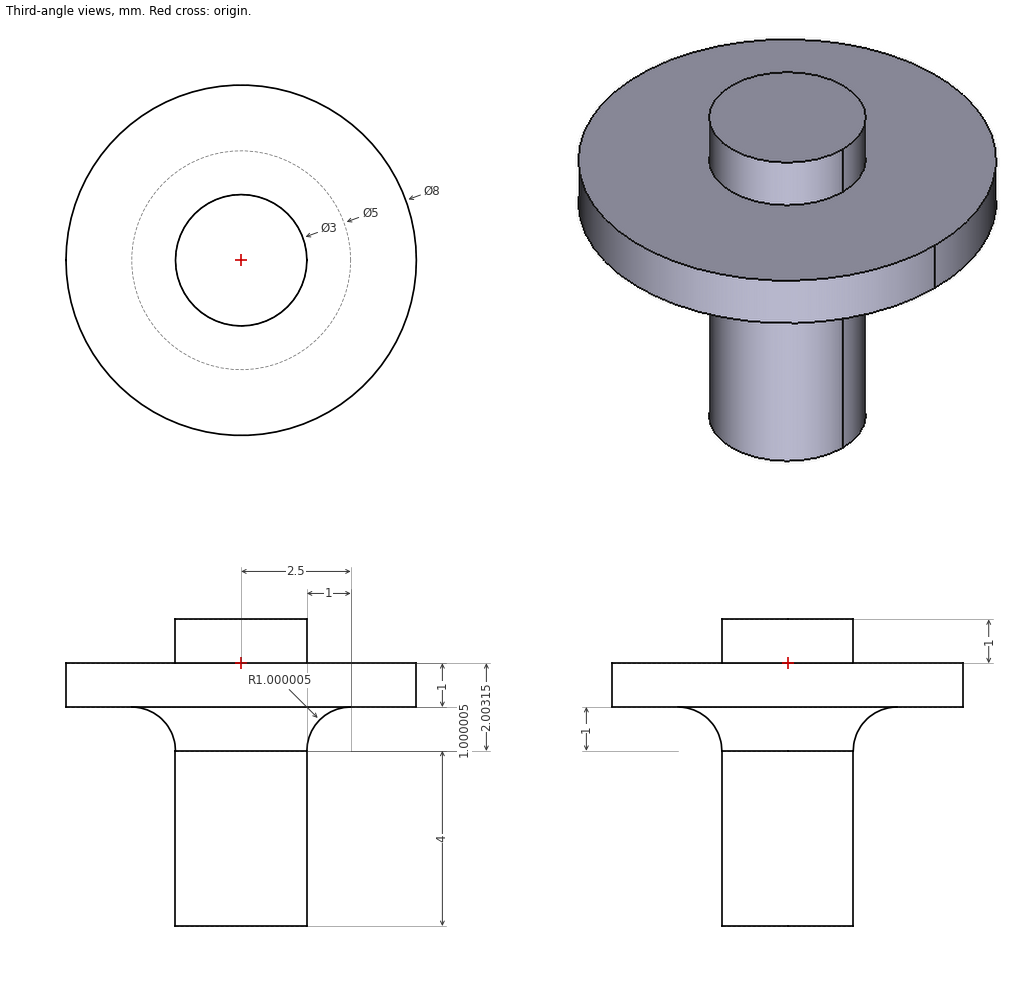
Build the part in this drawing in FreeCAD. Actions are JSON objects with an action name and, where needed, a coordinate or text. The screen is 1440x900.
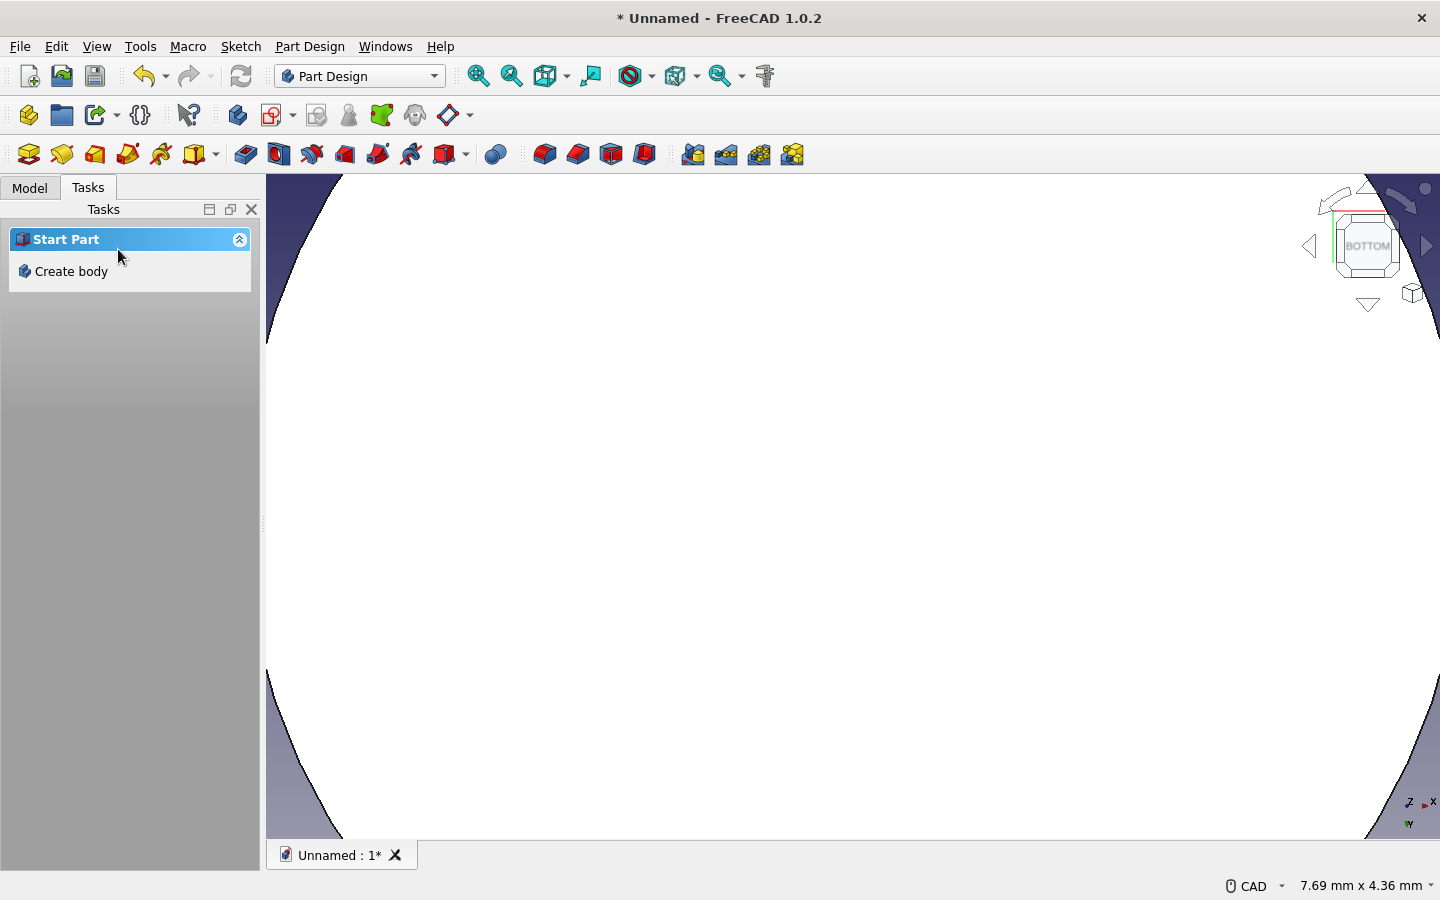
{"action": "left_click", "coordinate": [479, 76]}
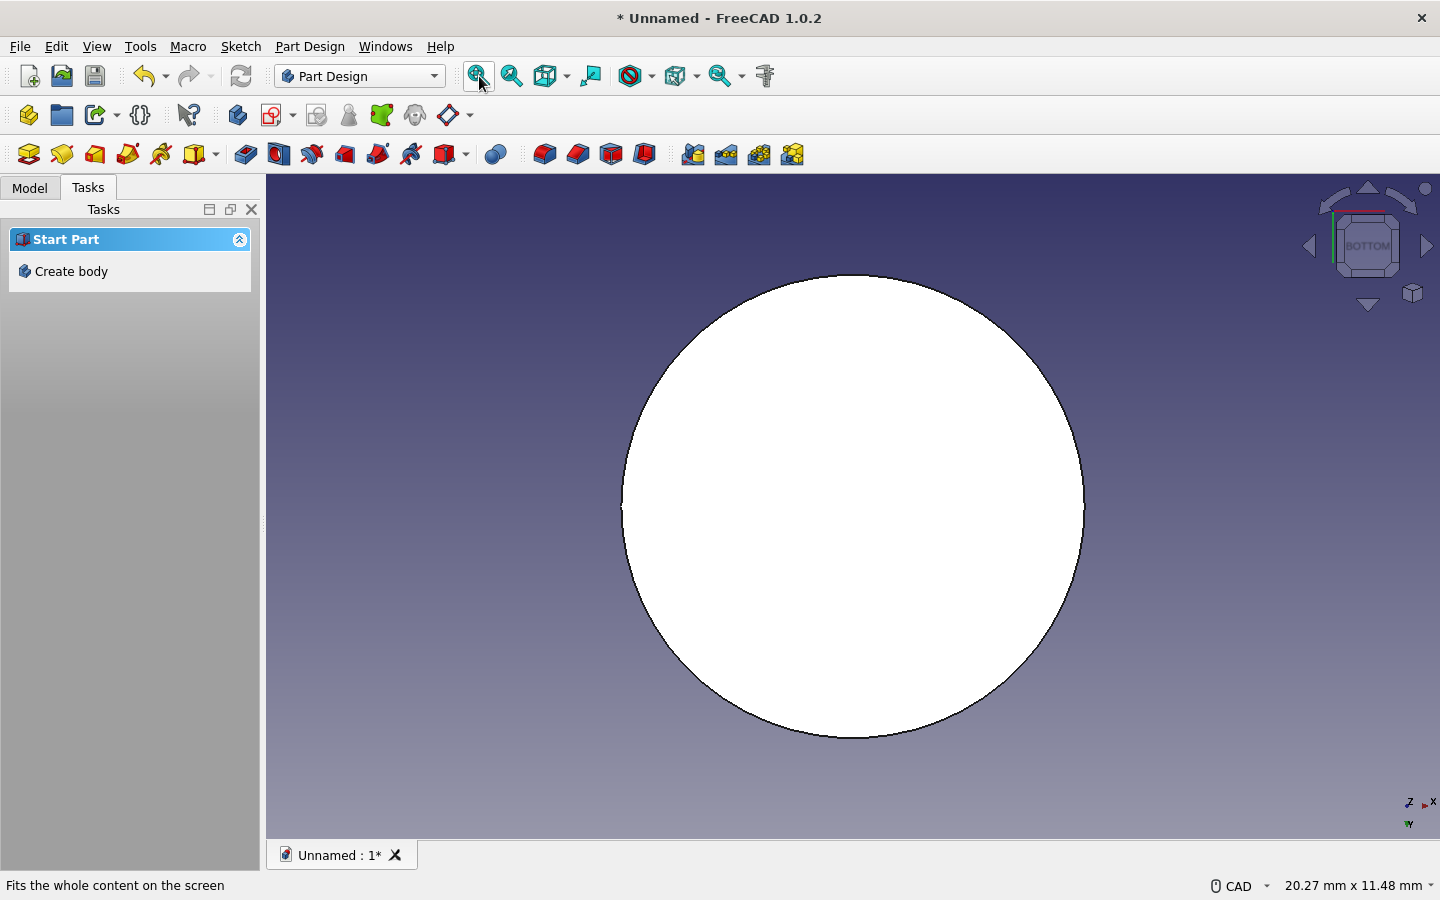
{"action": "left_click", "coordinate": [853, 505]}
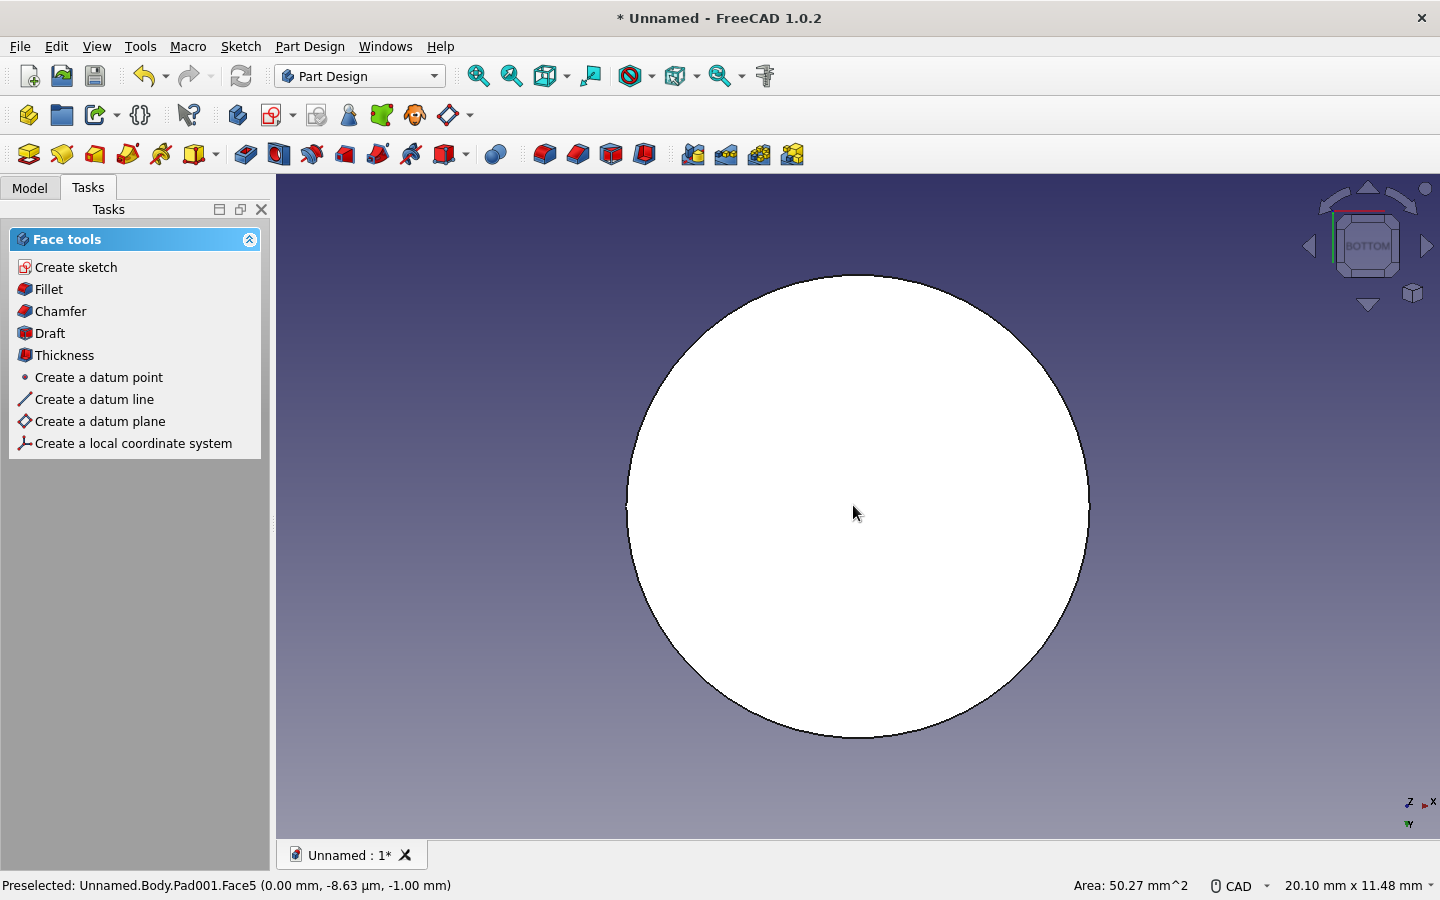
{"action": "left_click", "coordinate": [270, 116]}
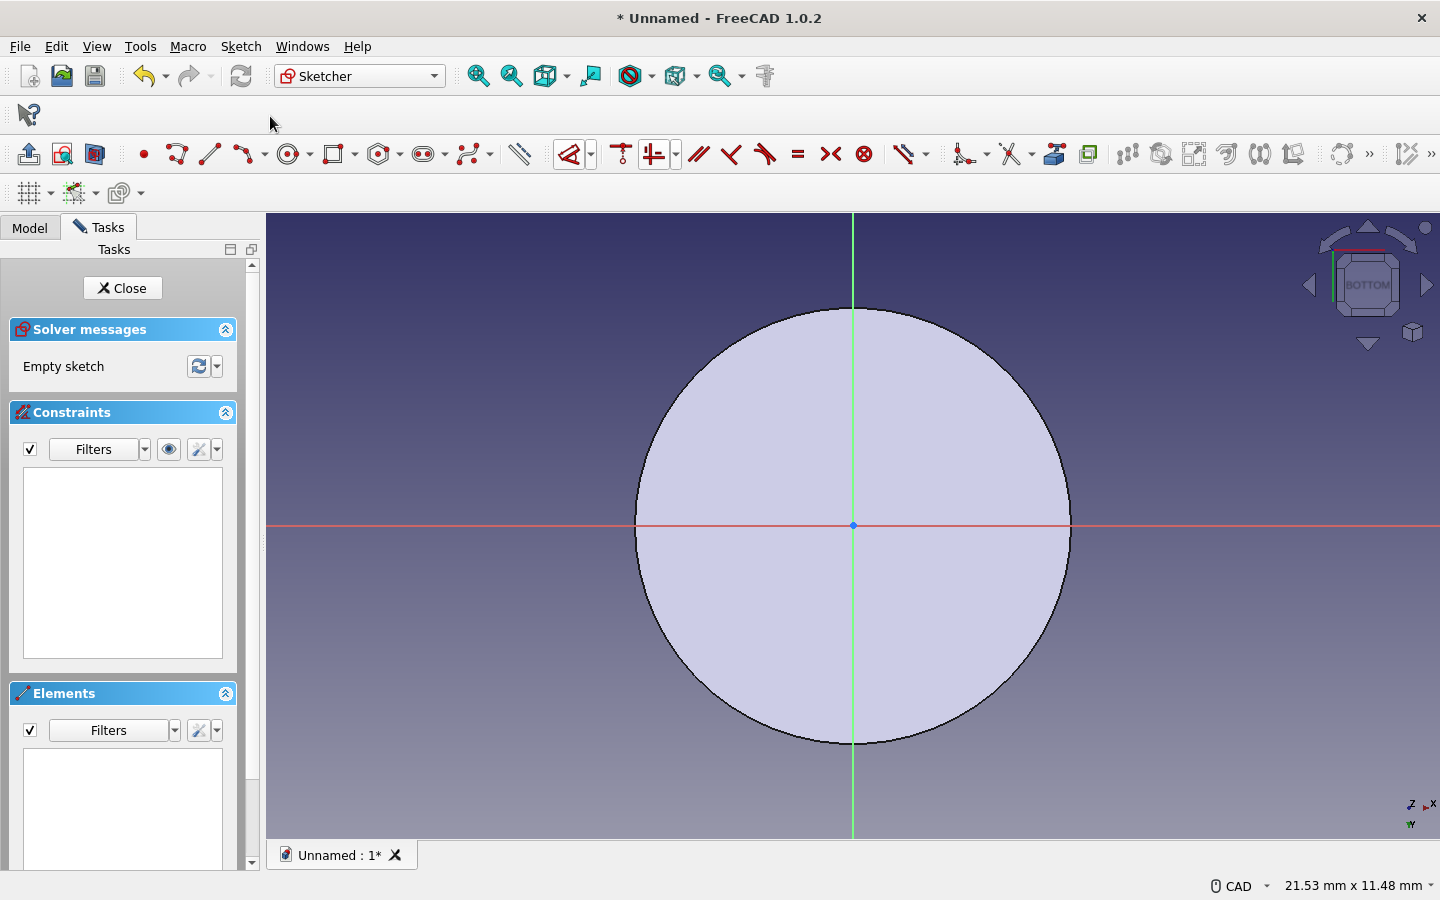
{"action": "scroll", "coordinate": [992, 526], "scroll_direction": "up", "scroll_amount": 2}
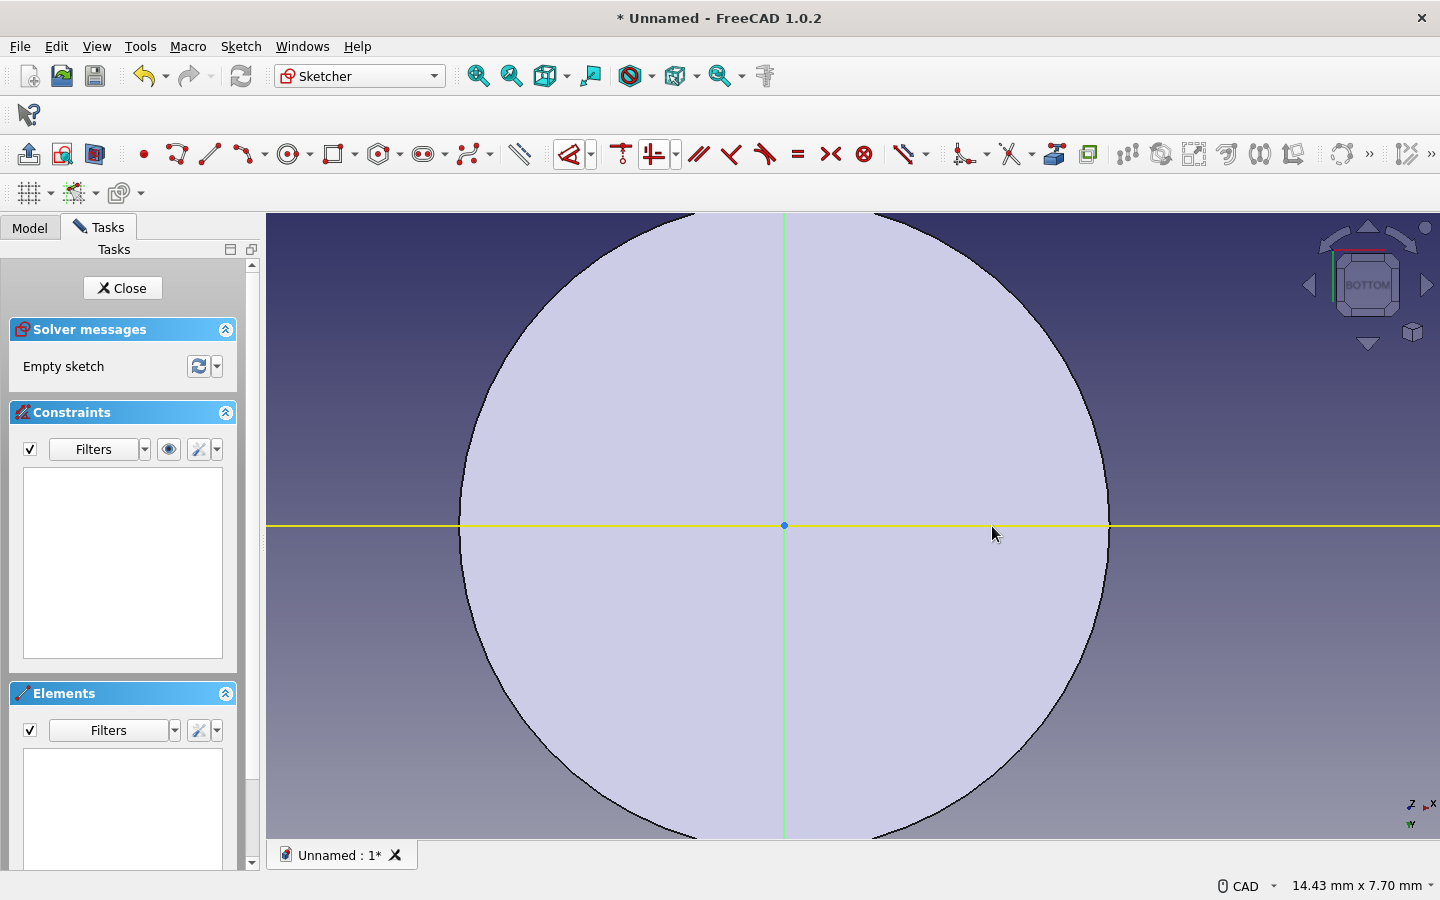
{"action": "left_click", "coordinate": [288, 154]}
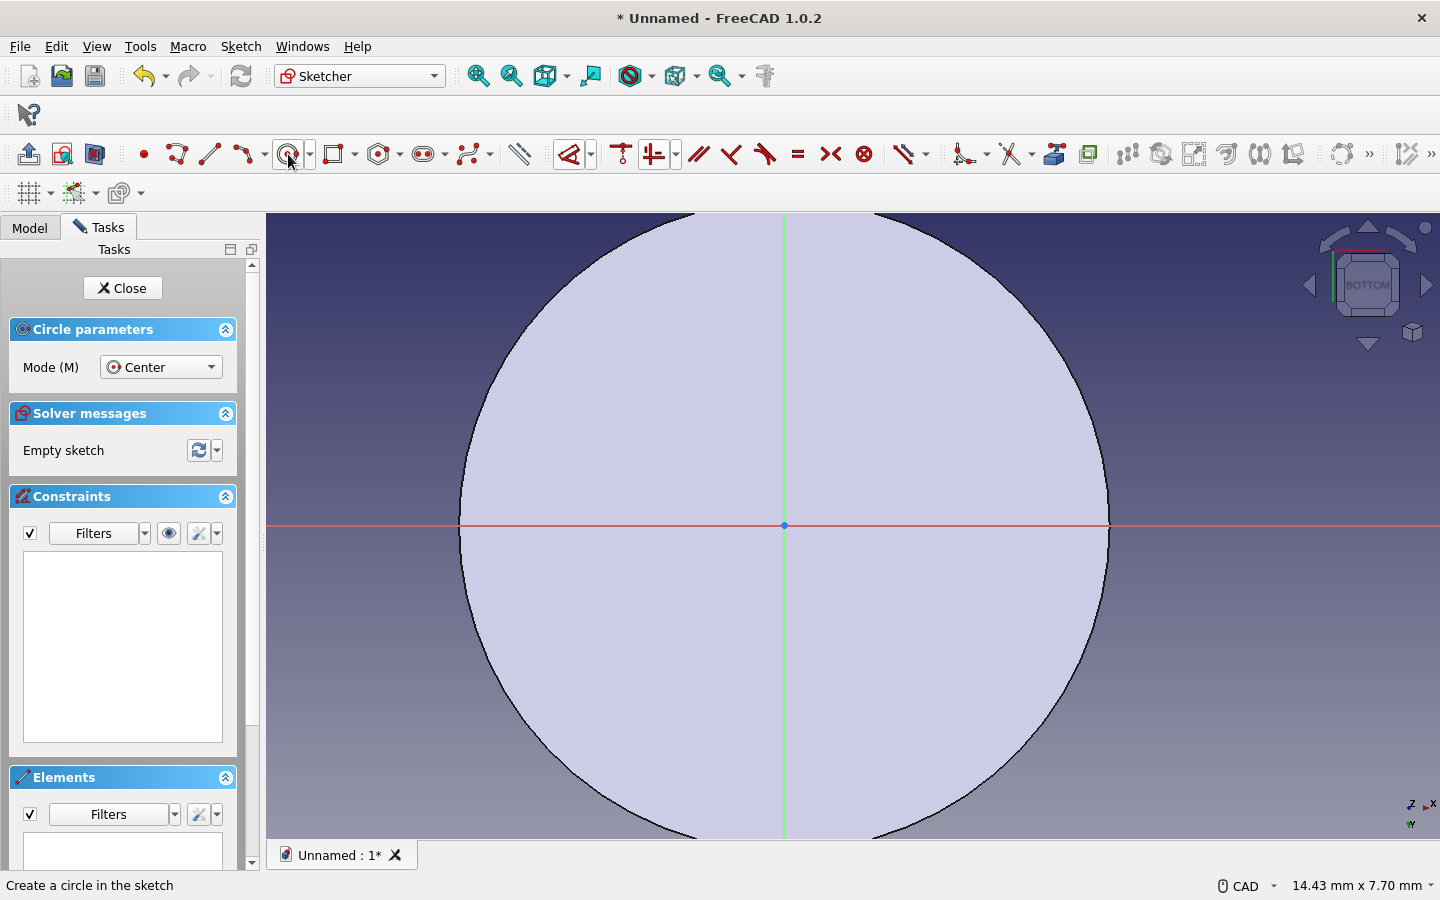
{"action": "left_click", "coordinate": [784, 526]}
{"action": "left_click", "coordinate": [928, 382]}
{"action": "key", "text": "Escape"}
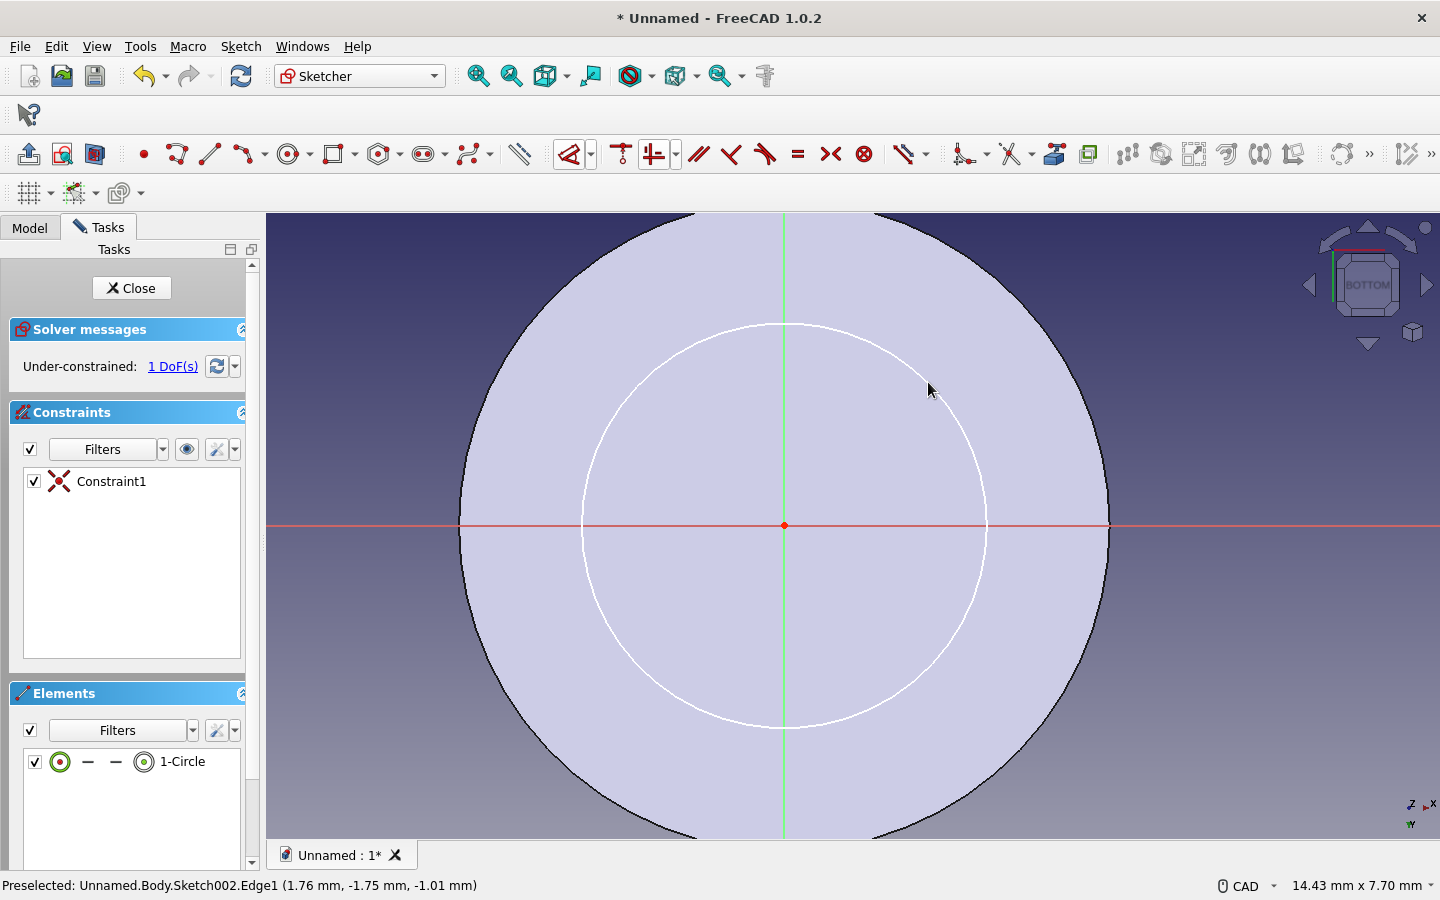
{"action": "left_click", "coordinate": [927, 382]}